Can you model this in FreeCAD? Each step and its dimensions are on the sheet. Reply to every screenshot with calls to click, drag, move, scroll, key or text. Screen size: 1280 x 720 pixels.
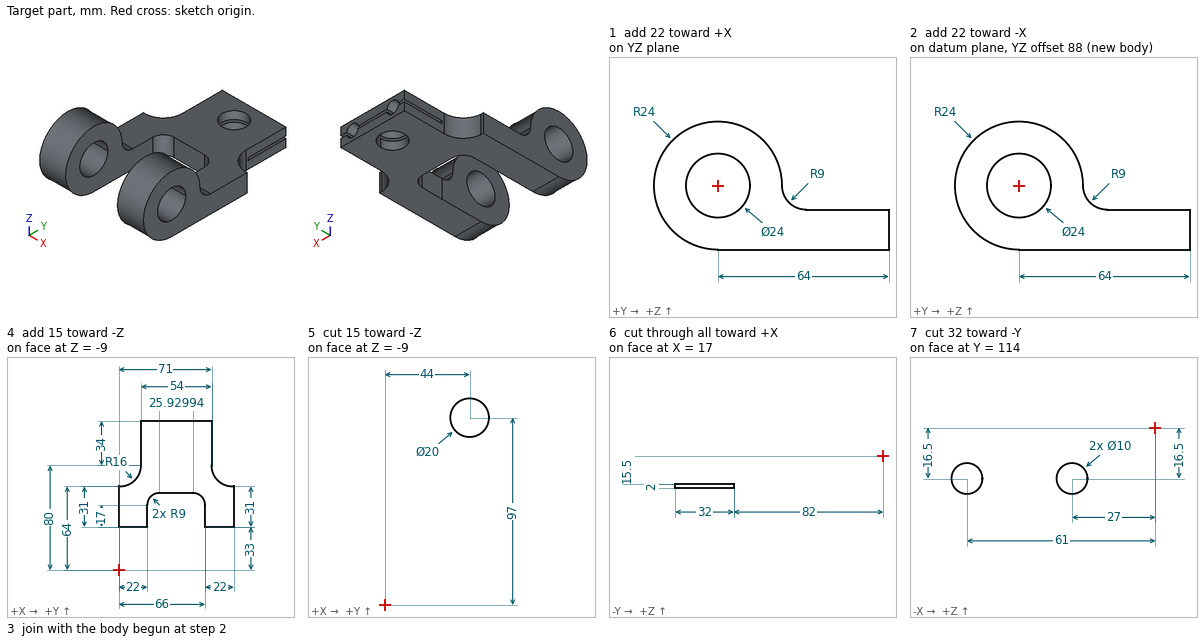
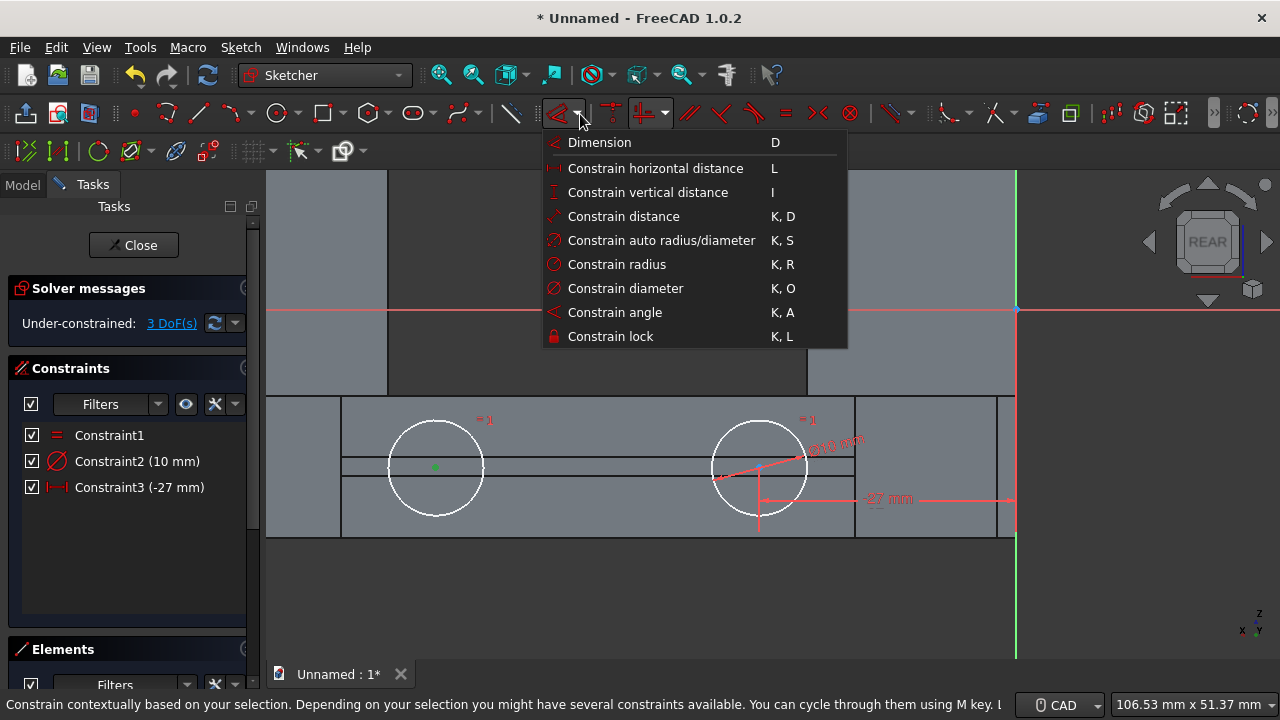
click(695, 168)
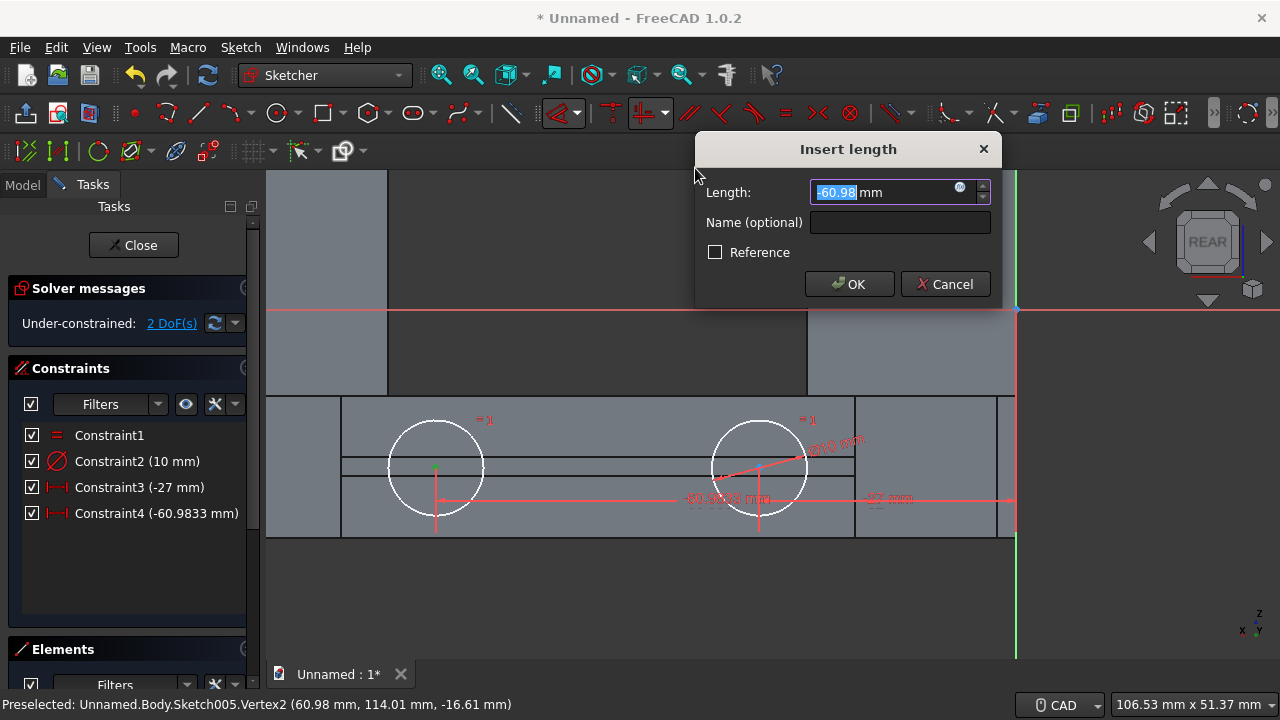
text(-61)
key(Return)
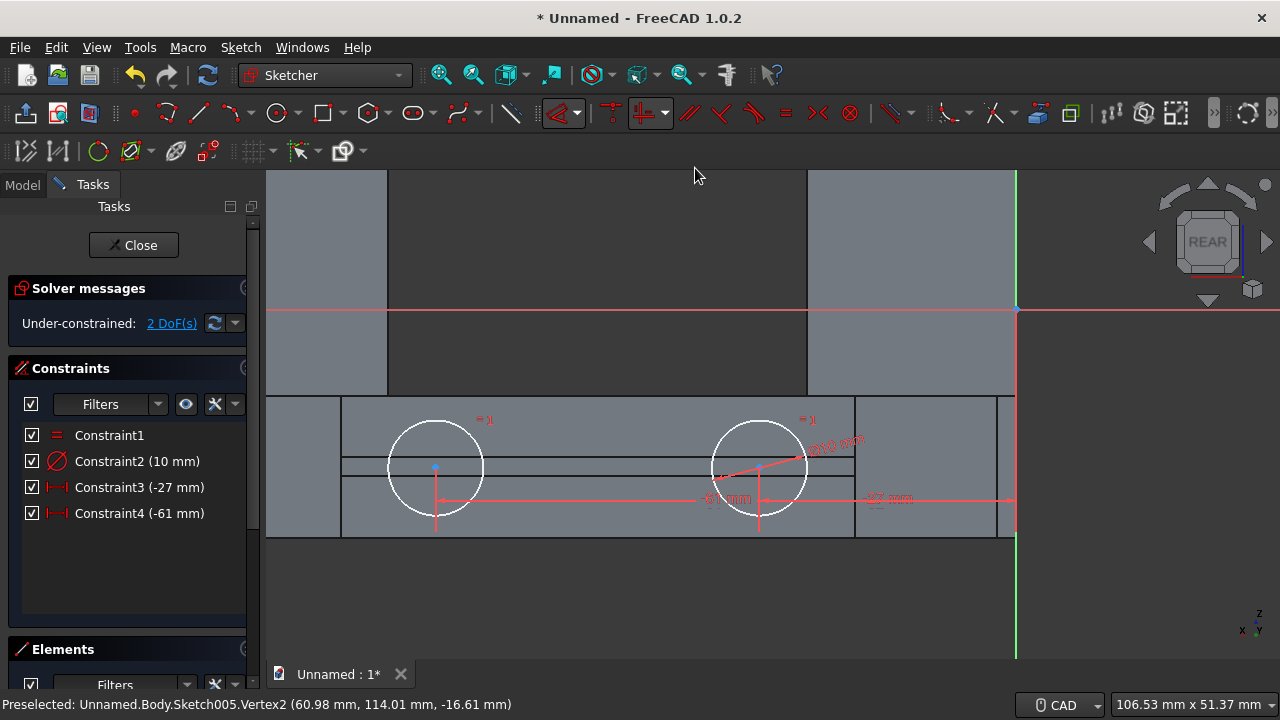
click(759, 468)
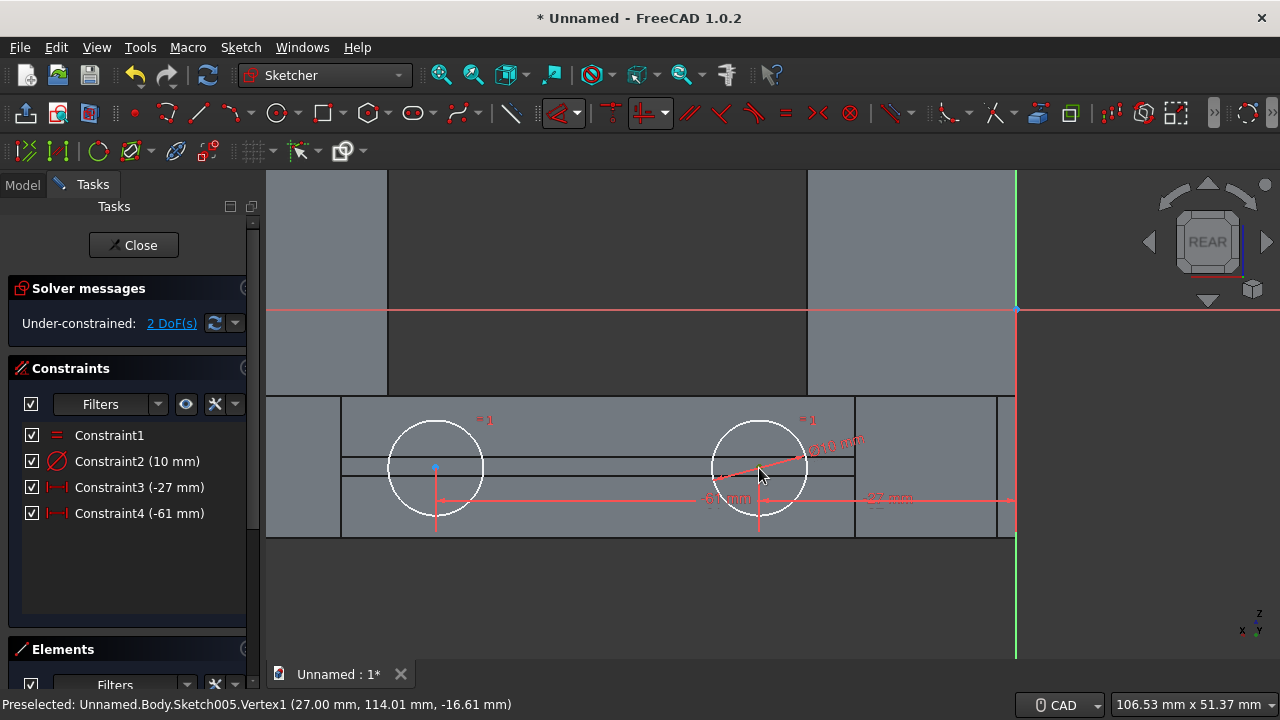
click(580, 114)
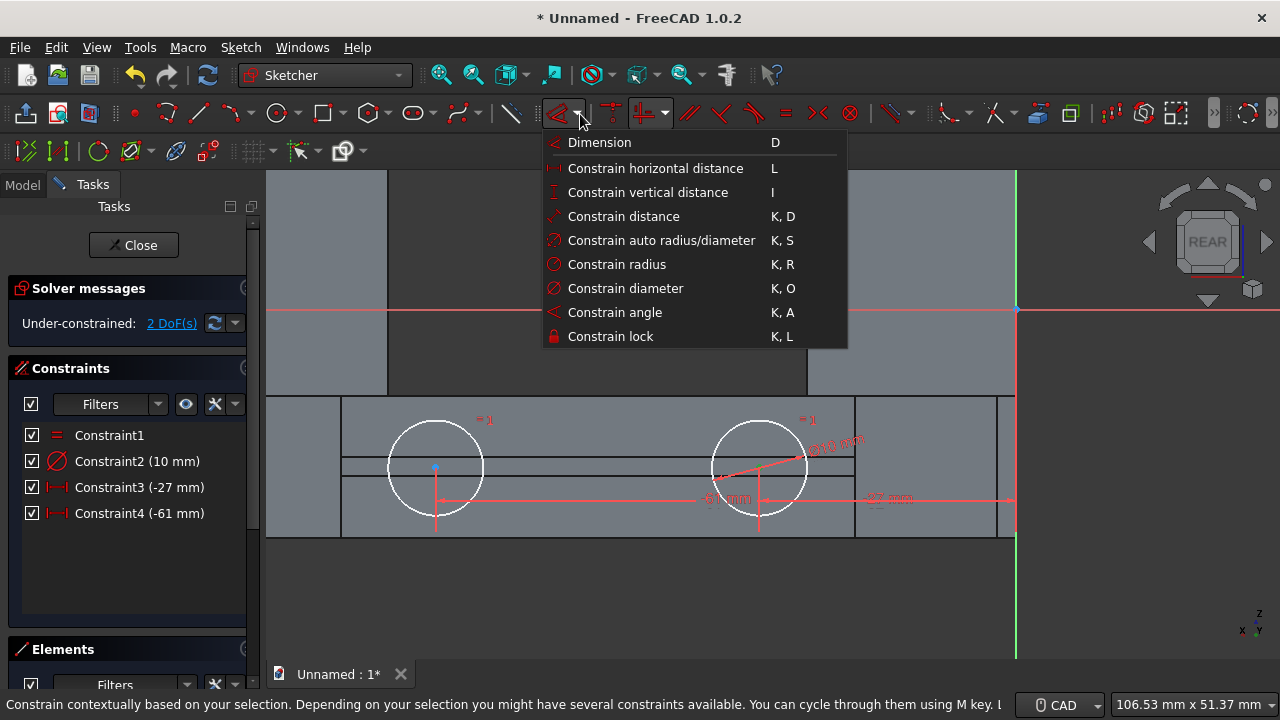
click(695, 192)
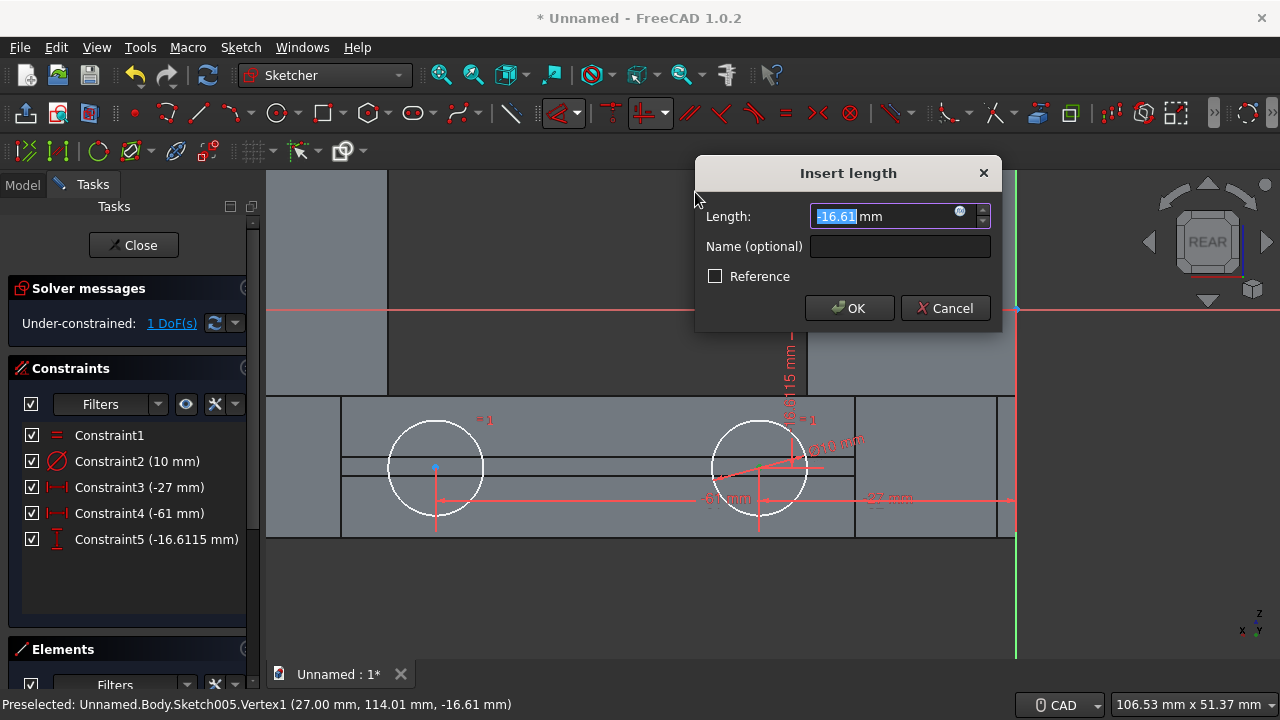
text(-16.5)
key(Return)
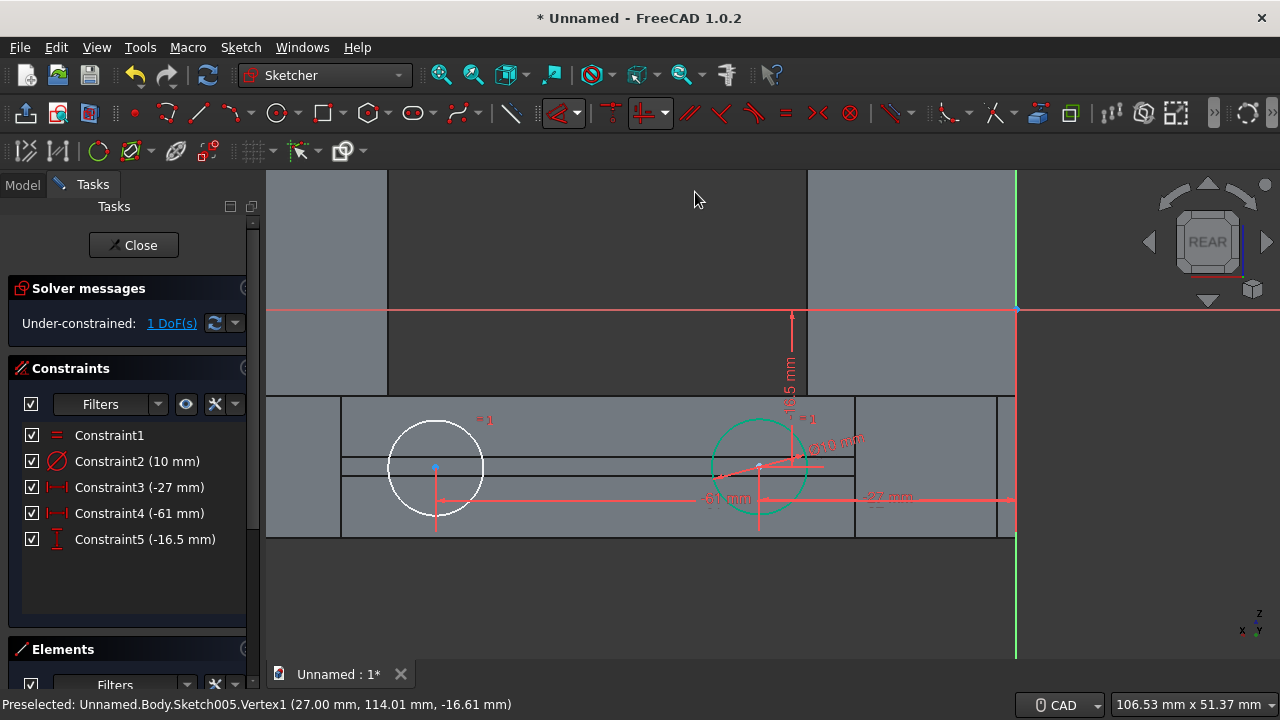
click(436, 468)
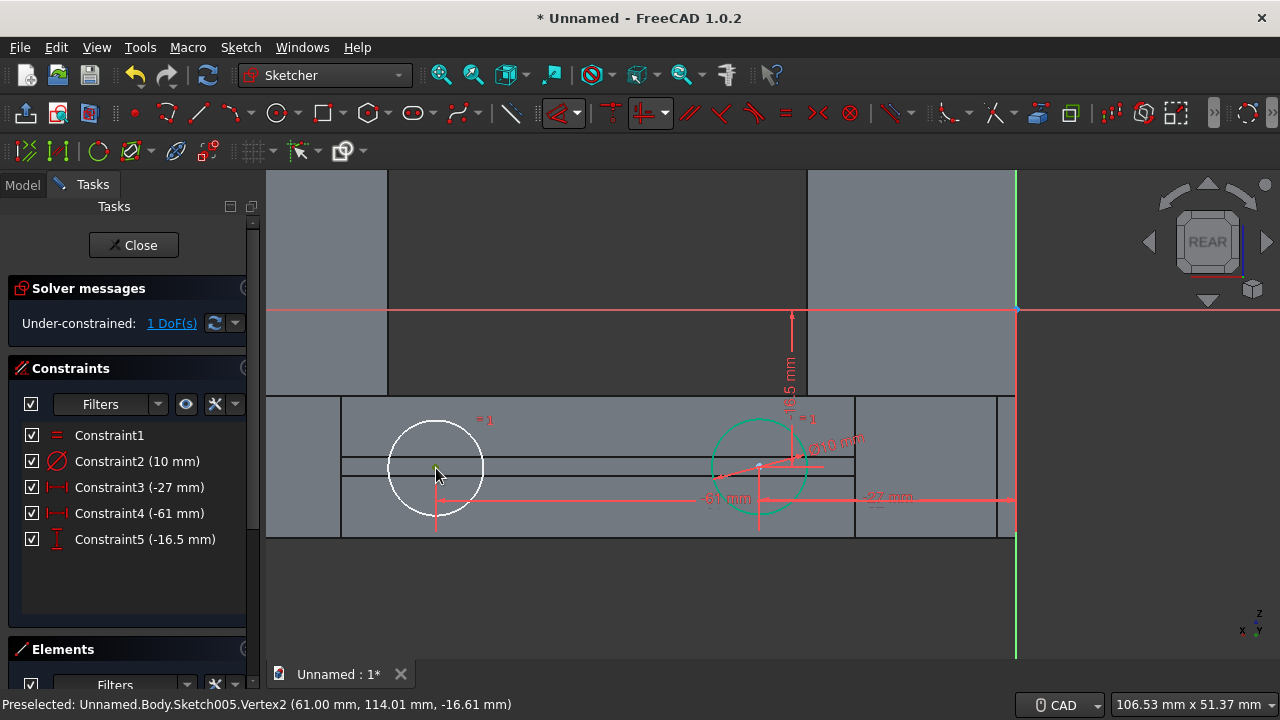
key(i)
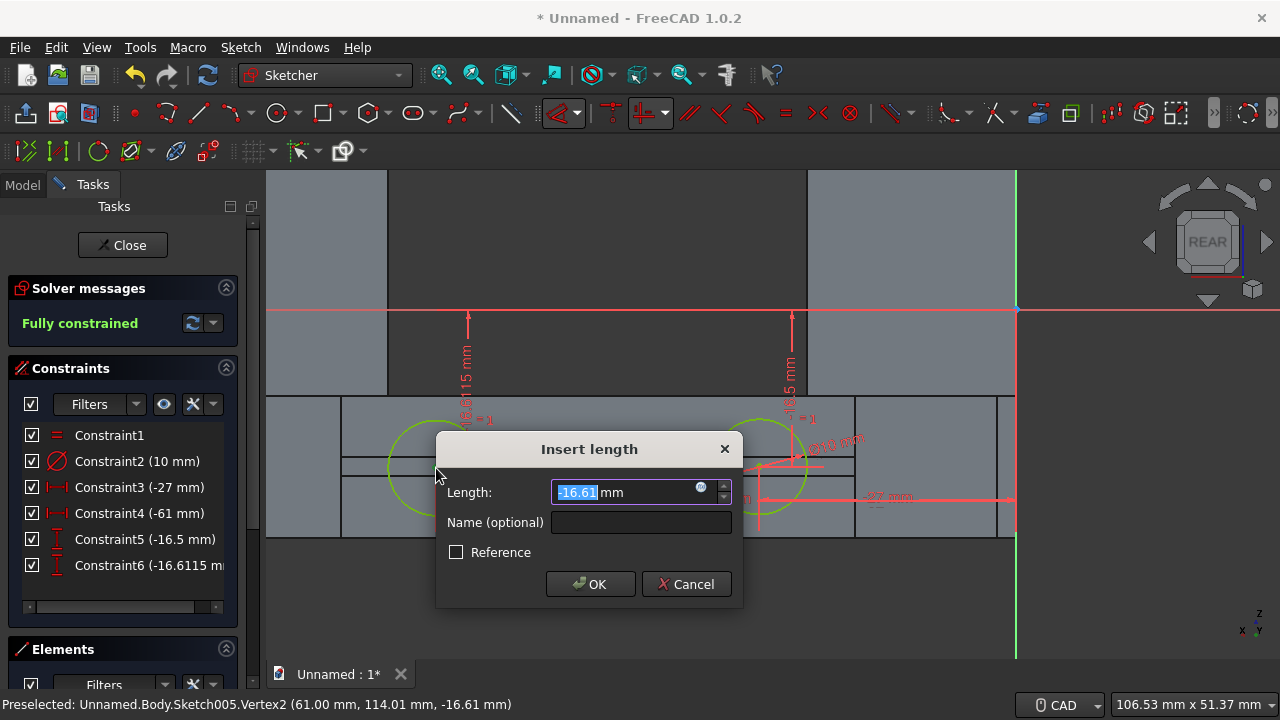
text(-16.5)
key(Return)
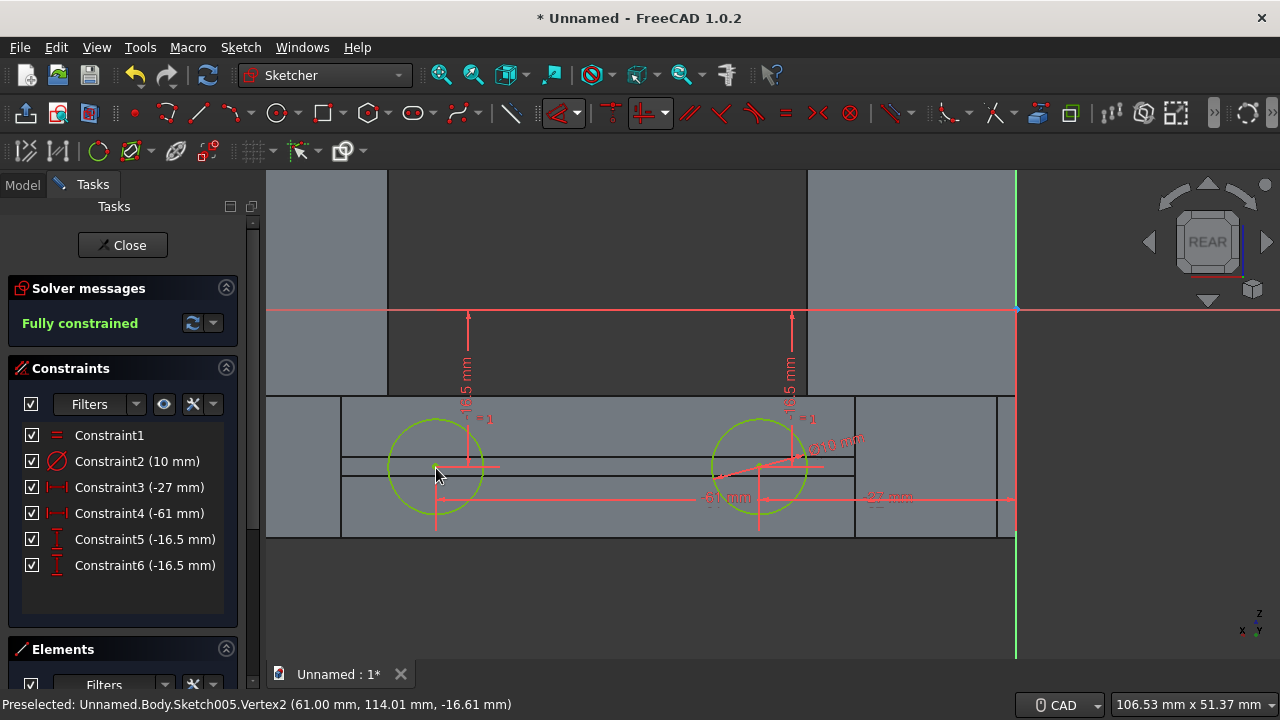
click(123, 245)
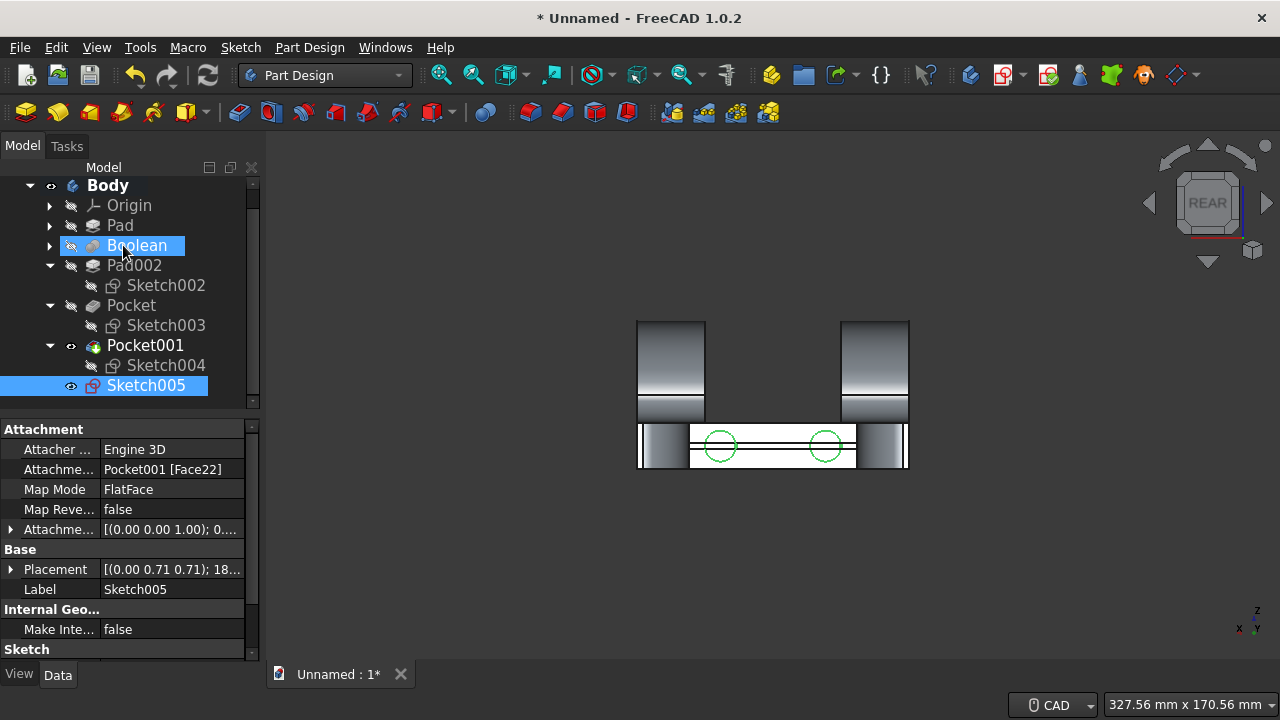
click(240, 112)